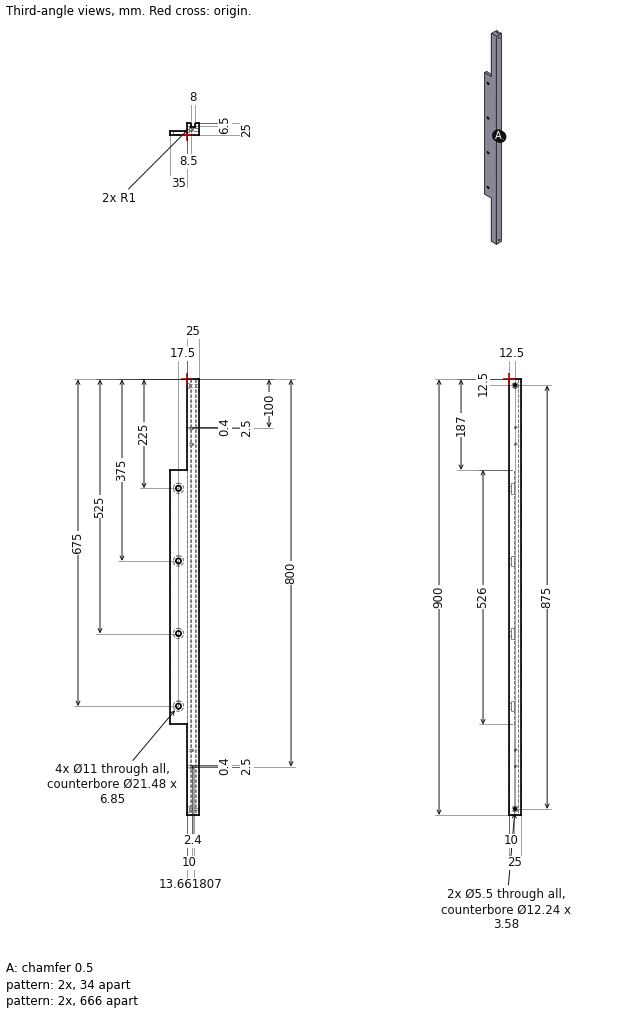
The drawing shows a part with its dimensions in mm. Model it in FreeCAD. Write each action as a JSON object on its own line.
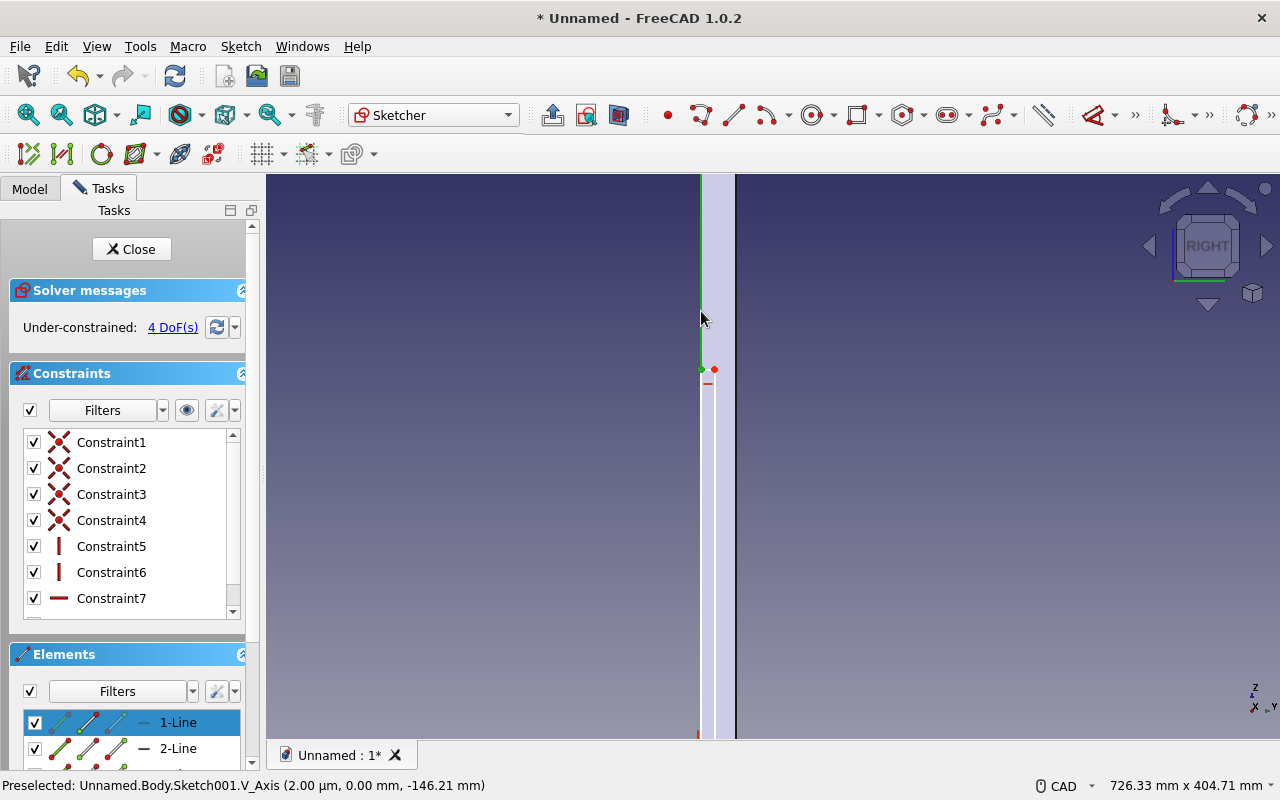
{"action": "key", "text": "c"}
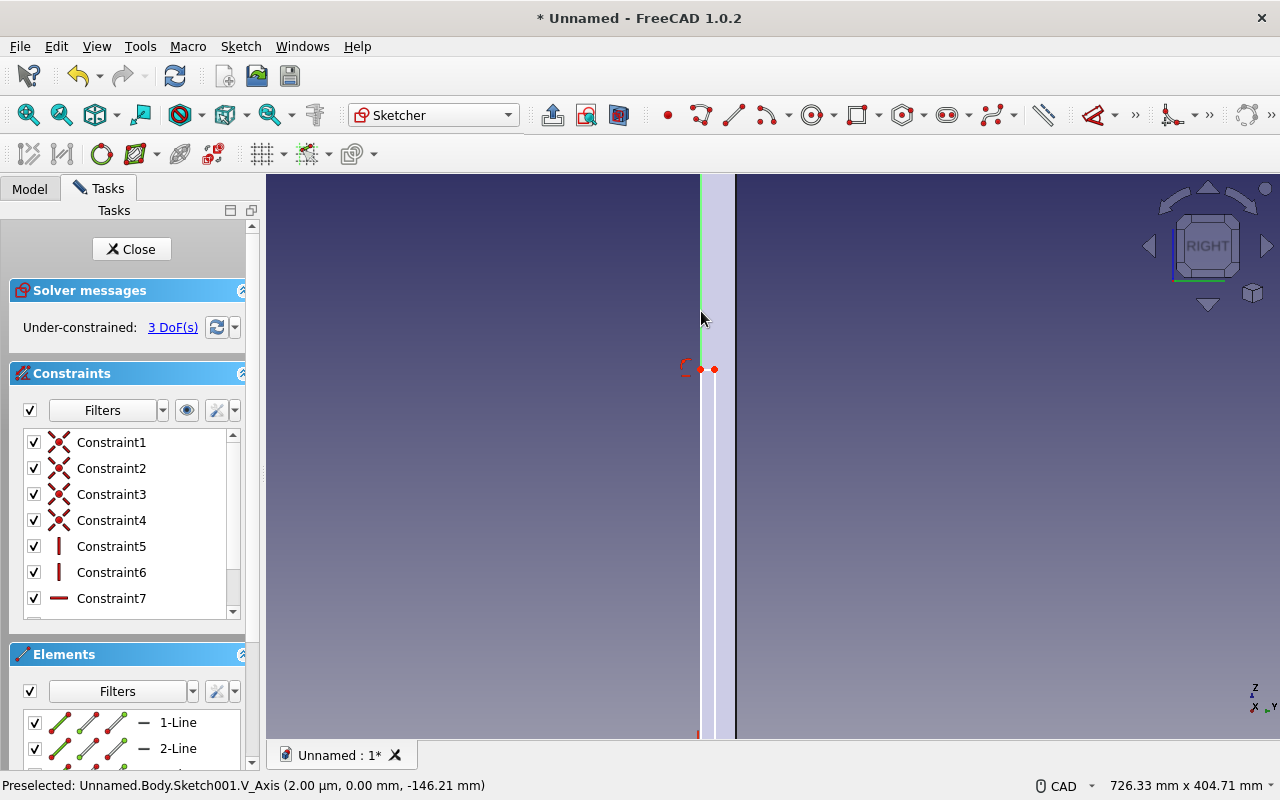
{"action": "scroll", "coordinate": [702, 370], "scroll_direction": "down", "scroll_amount": 5}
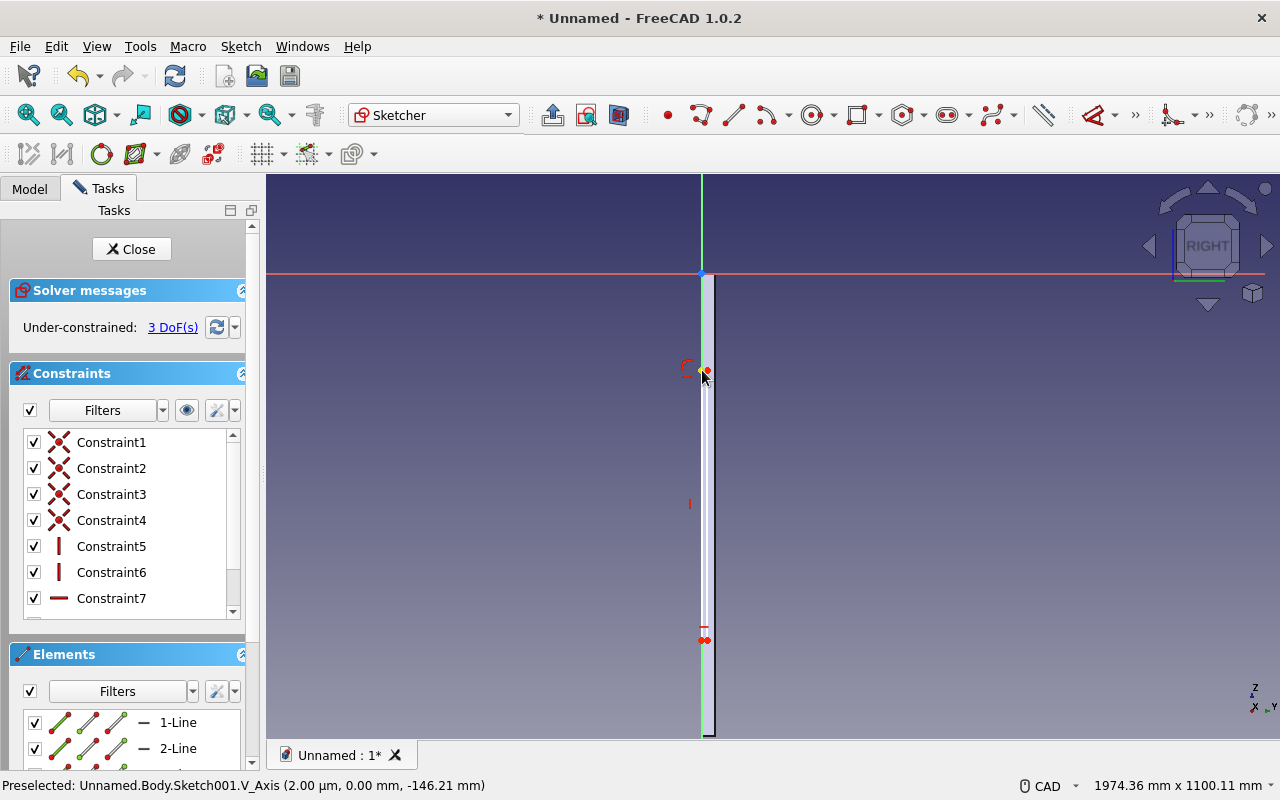
{"action": "scroll", "coordinate": [704, 640], "scroll_direction": "up", "scroll_amount": 11}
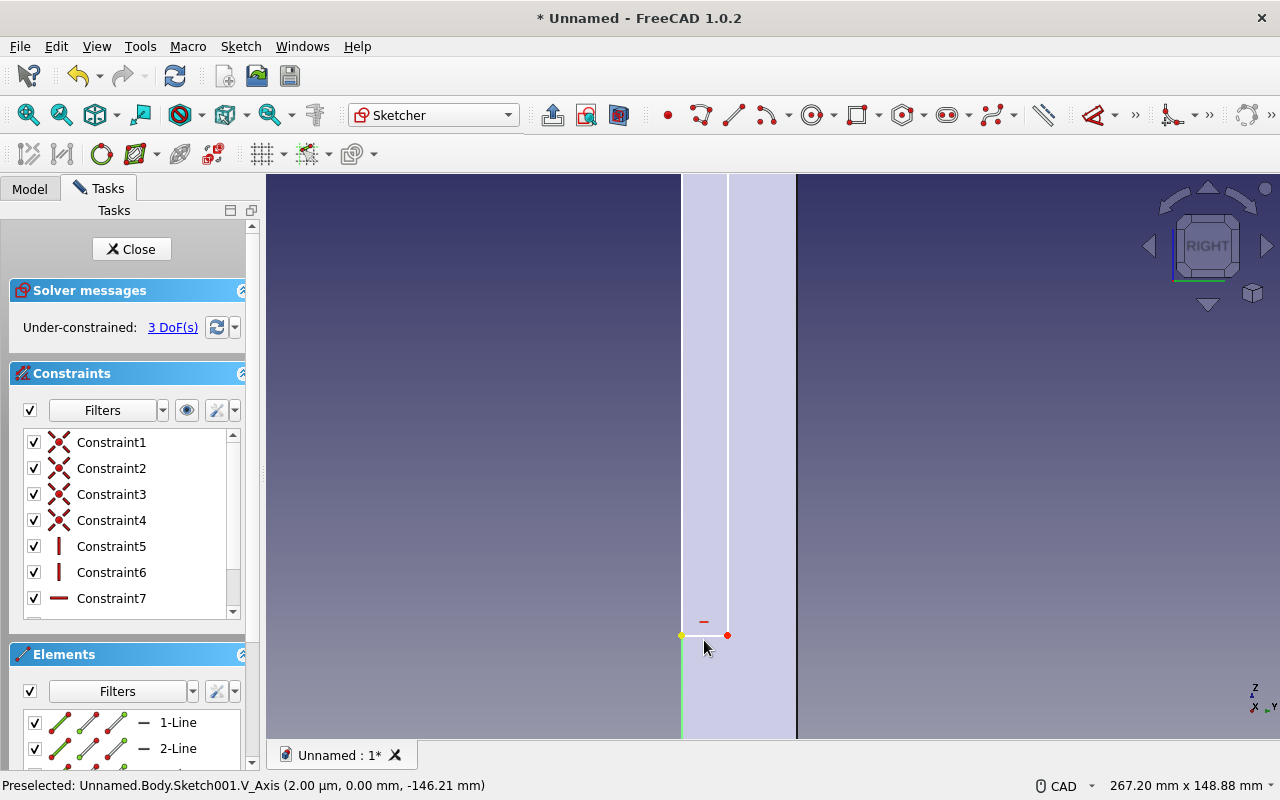
{"action": "left_click", "coordinate": [705, 636]}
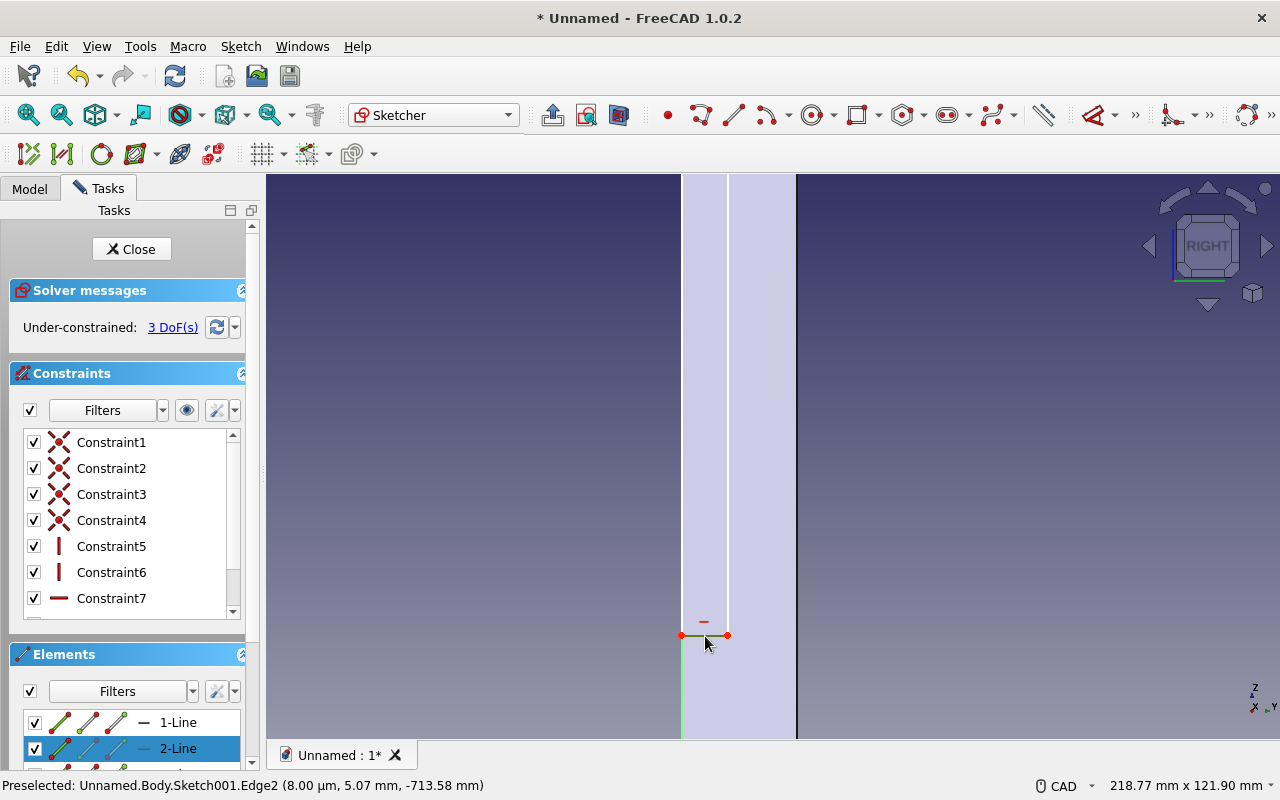
{"action": "left_click", "coordinate": [1114, 116]}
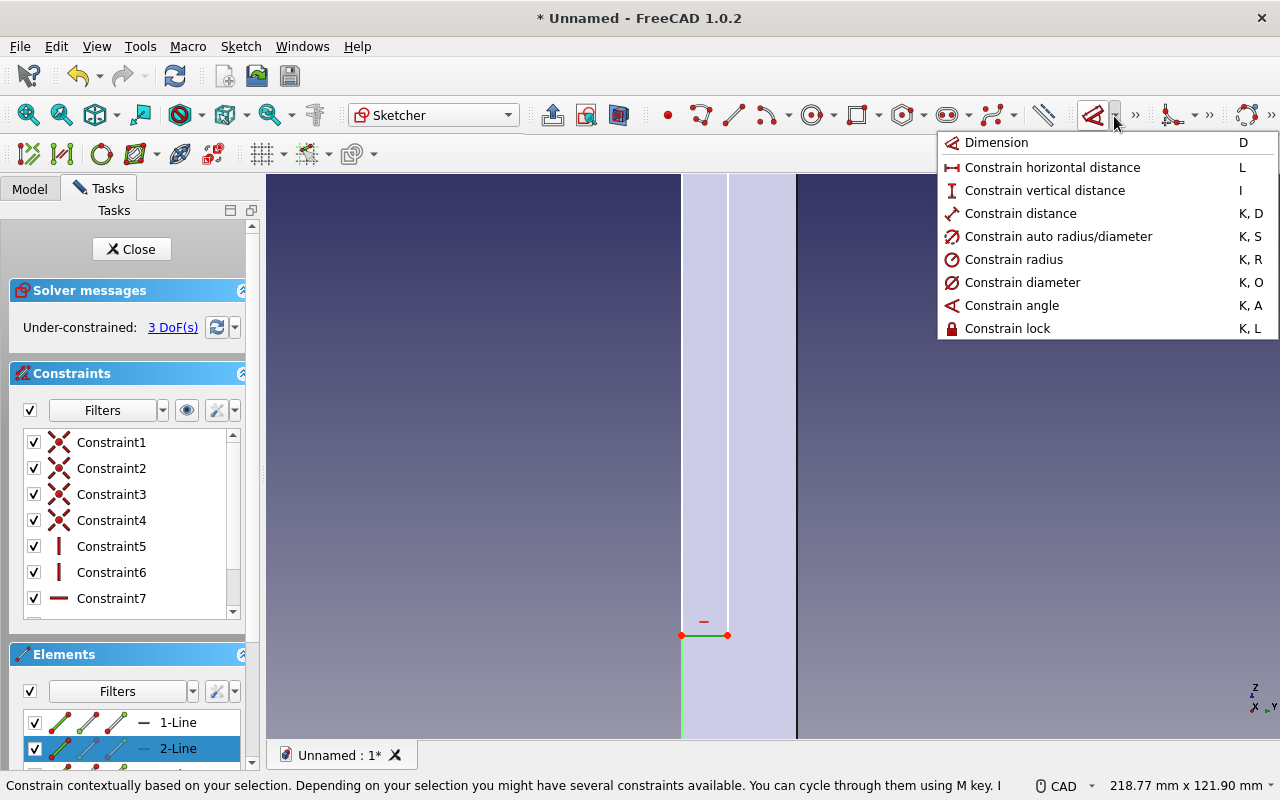
{"action": "left_click", "coordinate": [1108, 168]}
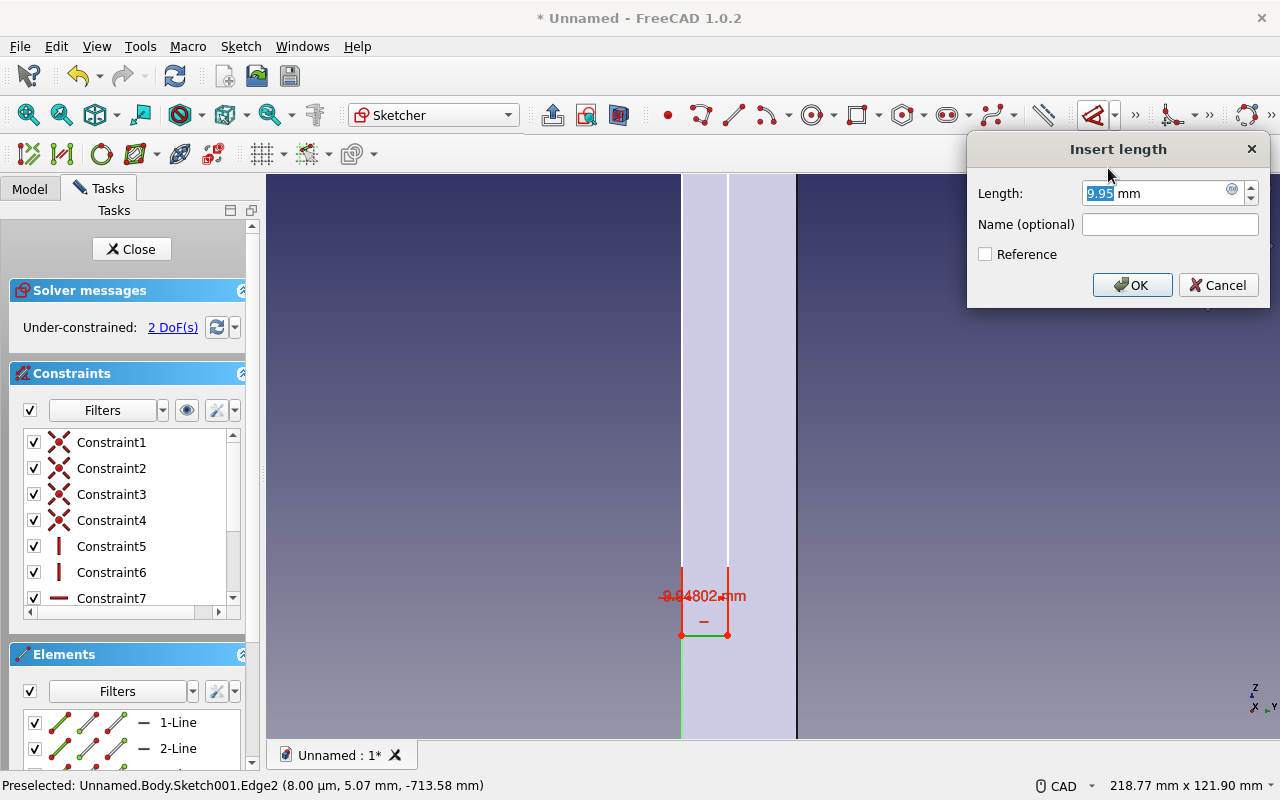
{"action": "type", "text": "10"}
{"action": "key", "text": "Return"}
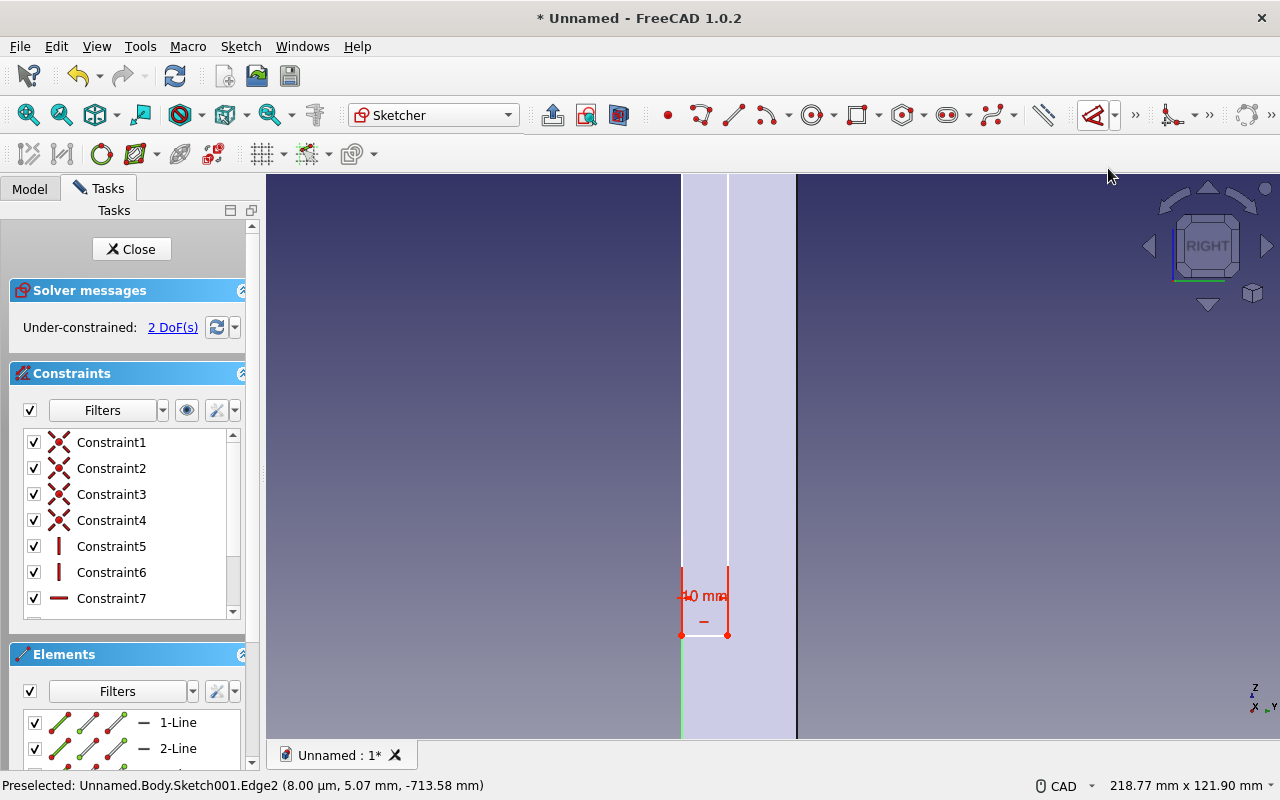
{"action": "scroll", "coordinate": [704, 640], "scroll_direction": "down", "scroll_amount": 11}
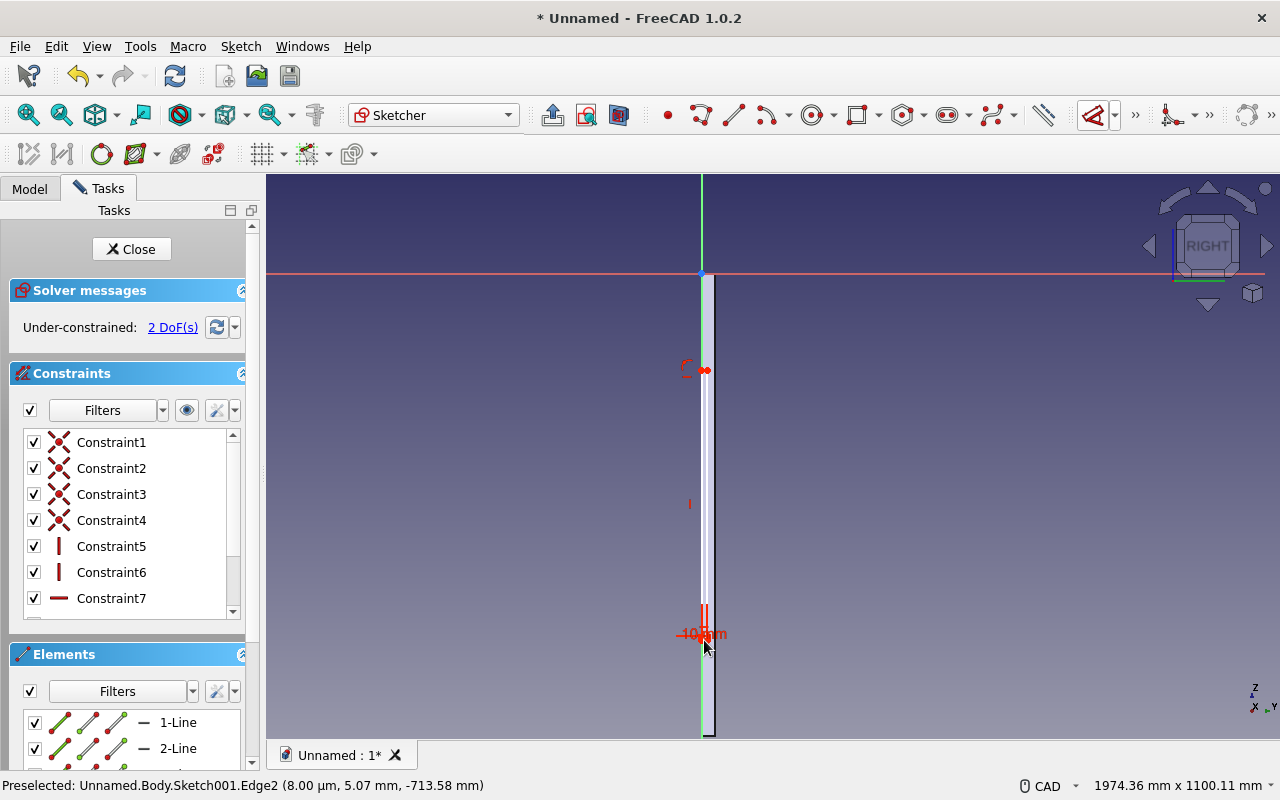
{"action": "scroll", "coordinate": [702, 451], "scroll_direction": "up", "scroll_amount": 5}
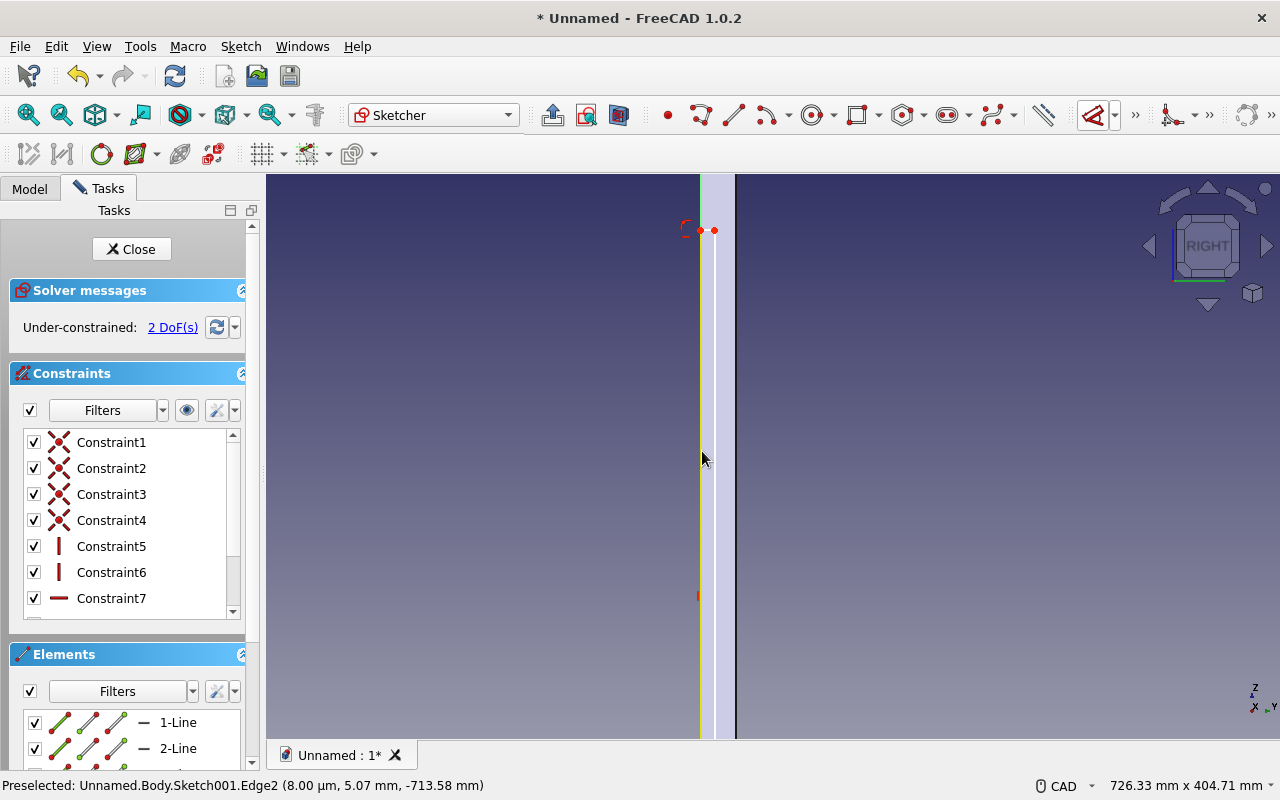
{"action": "left_click", "coordinate": [701, 450]}